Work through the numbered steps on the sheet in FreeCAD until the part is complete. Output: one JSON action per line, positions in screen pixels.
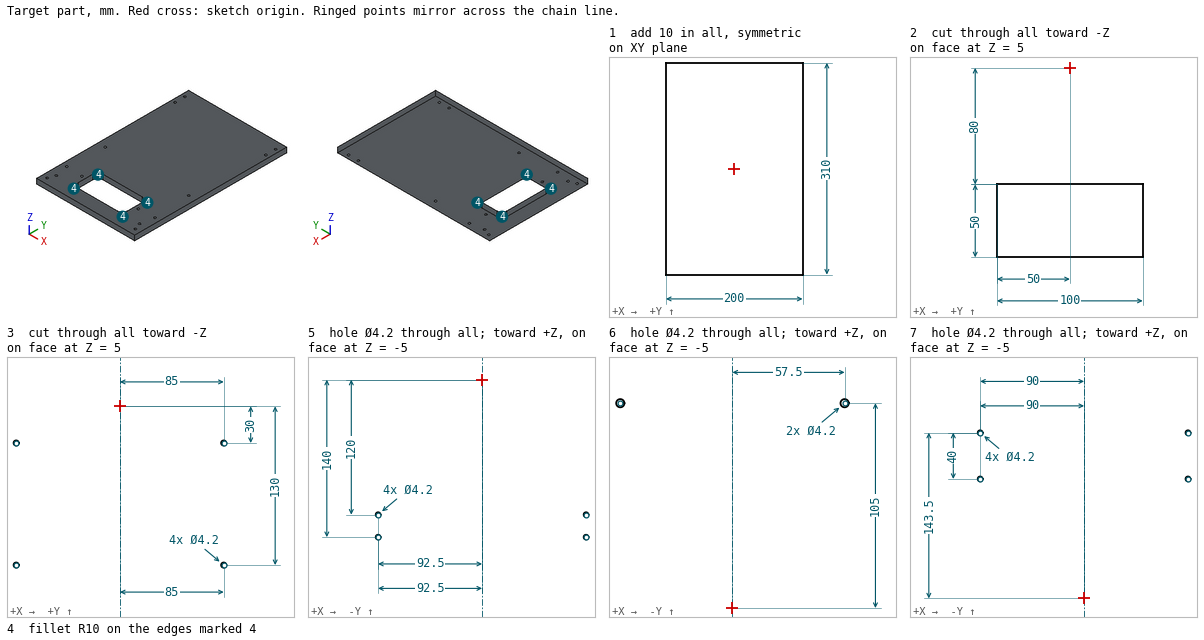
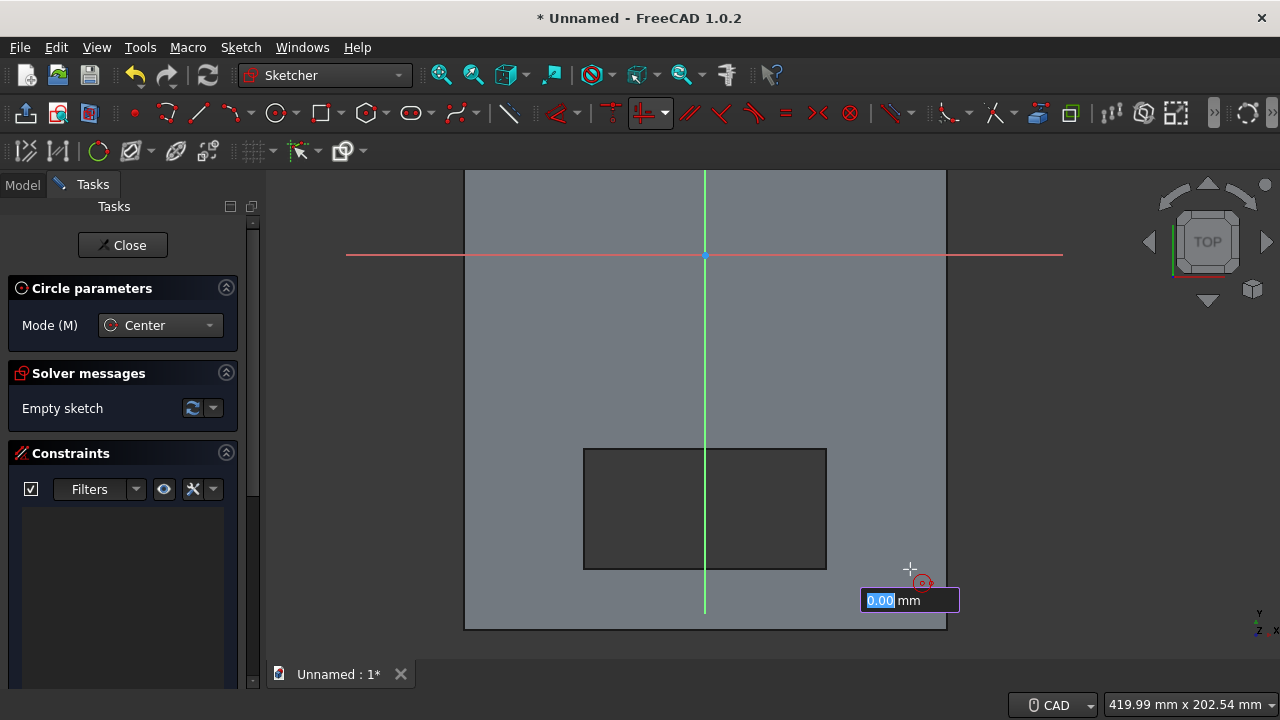
{"action": "scroll", "coordinate": [914, 566], "scroll_direction": "up", "scroll_amount": 6}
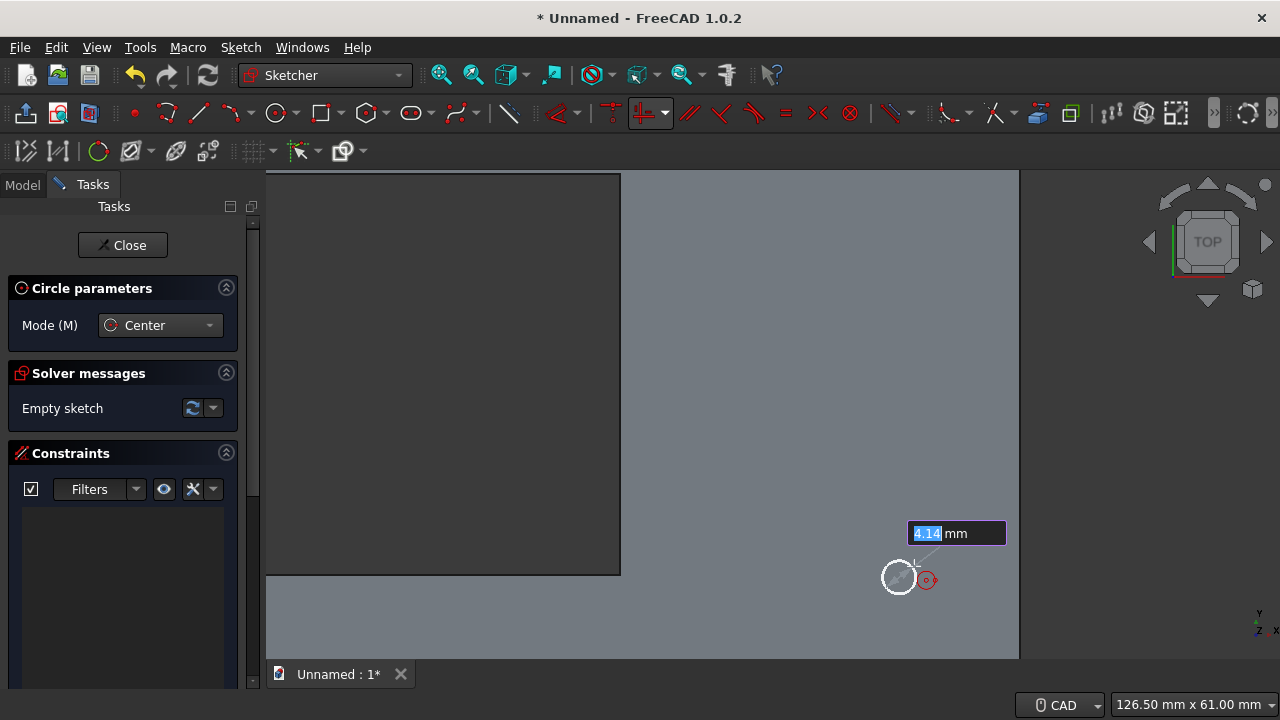
{"action": "left_click", "coordinate": [912, 563]}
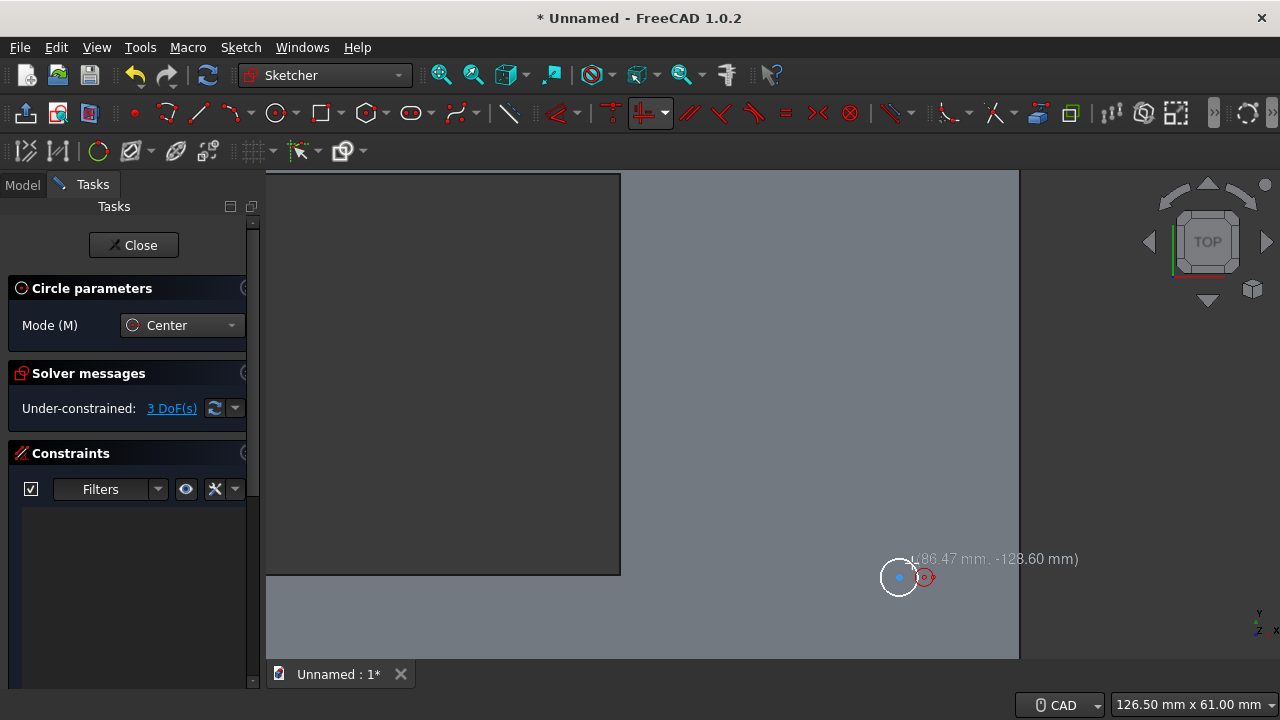
{"action": "scroll", "coordinate": [914, 566], "scroll_direction": "down", "scroll_amount": 6}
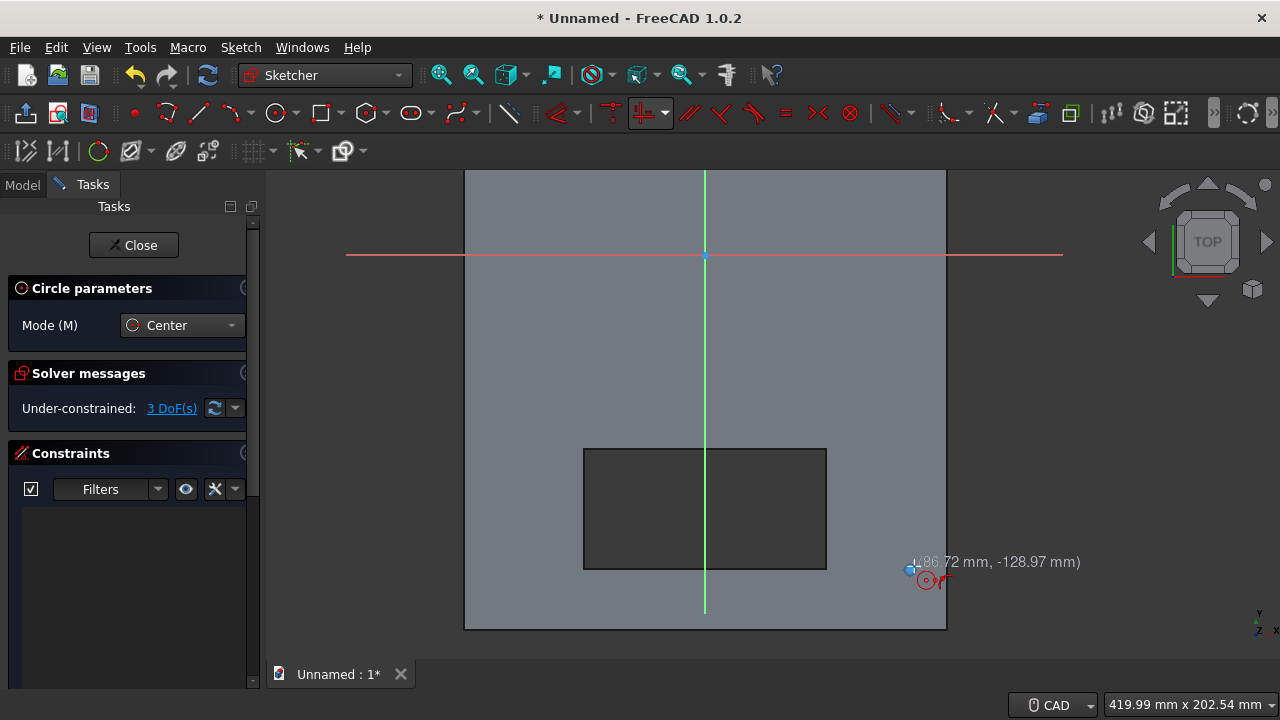
{"action": "scroll", "coordinate": [910, 328], "scroll_direction": "up", "scroll_amount": 8}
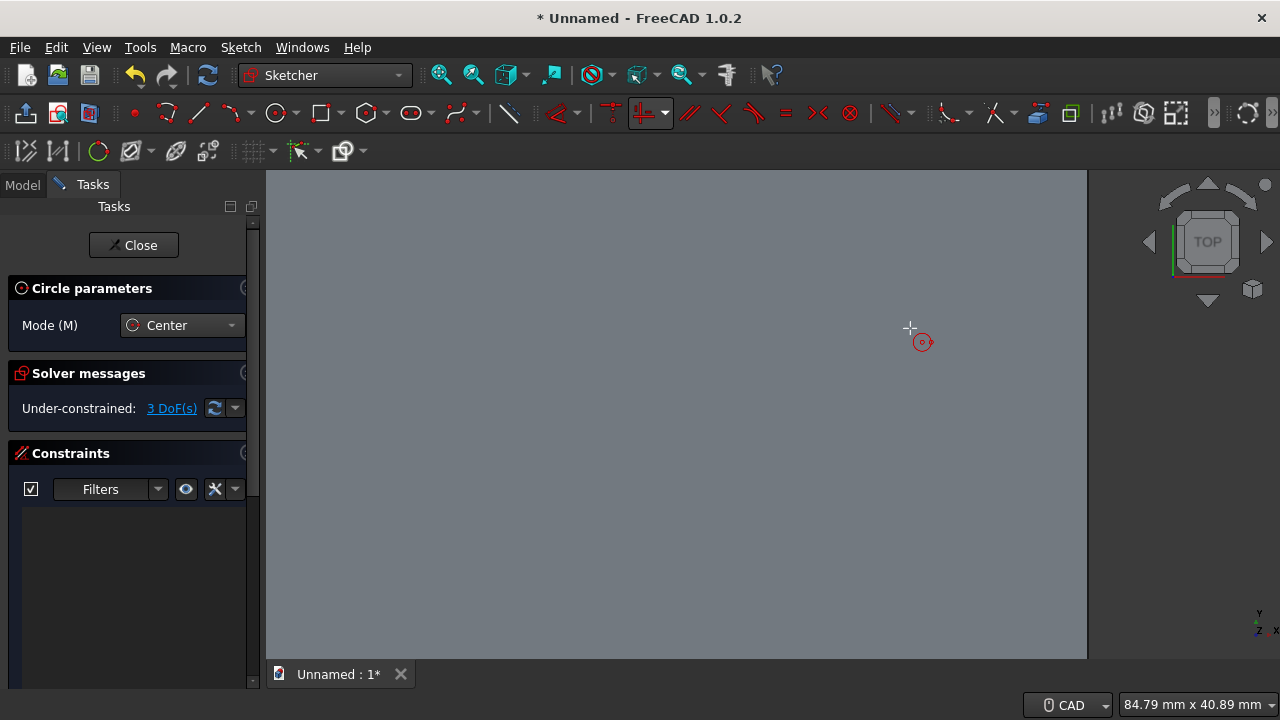
{"action": "scroll", "coordinate": [910, 328], "scroll_direction": "down", "scroll_amount": 8}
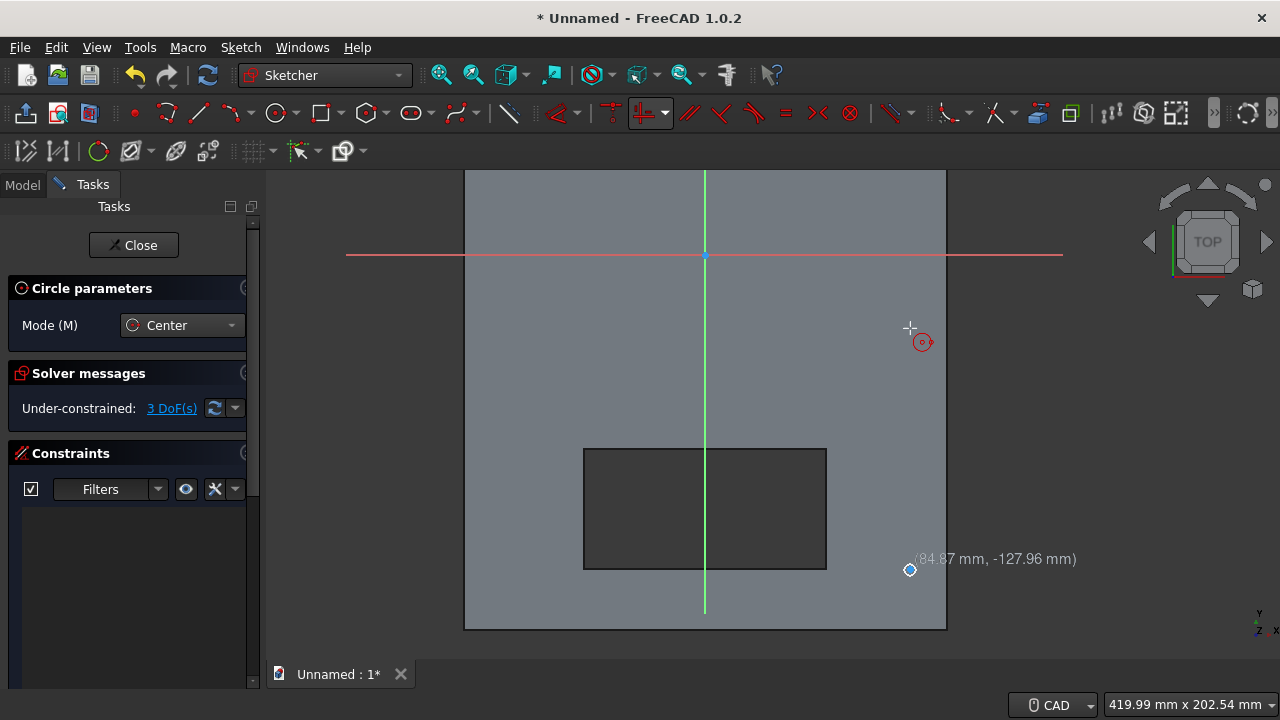
{"action": "left_click", "coordinate": [910, 328]}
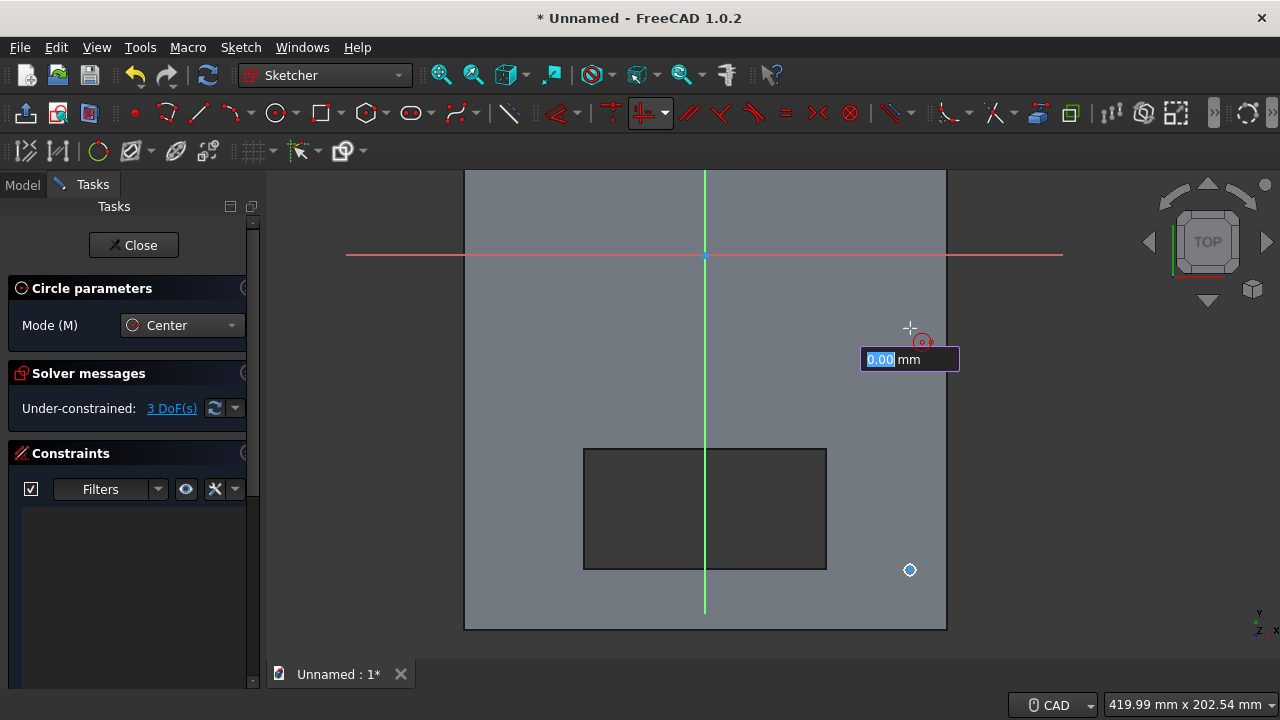
{"action": "scroll", "coordinate": [914, 324], "scroll_direction": "up", "scroll_amount": 6}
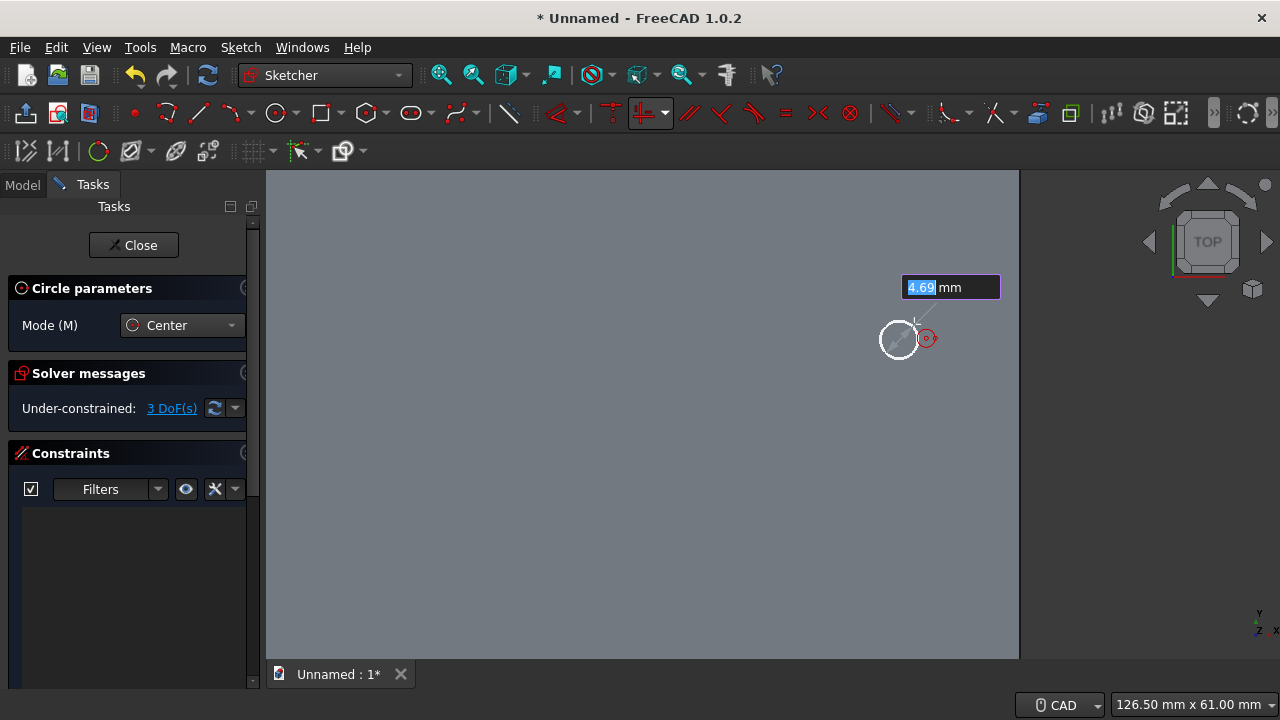
{"action": "left_click", "coordinate": [912, 324]}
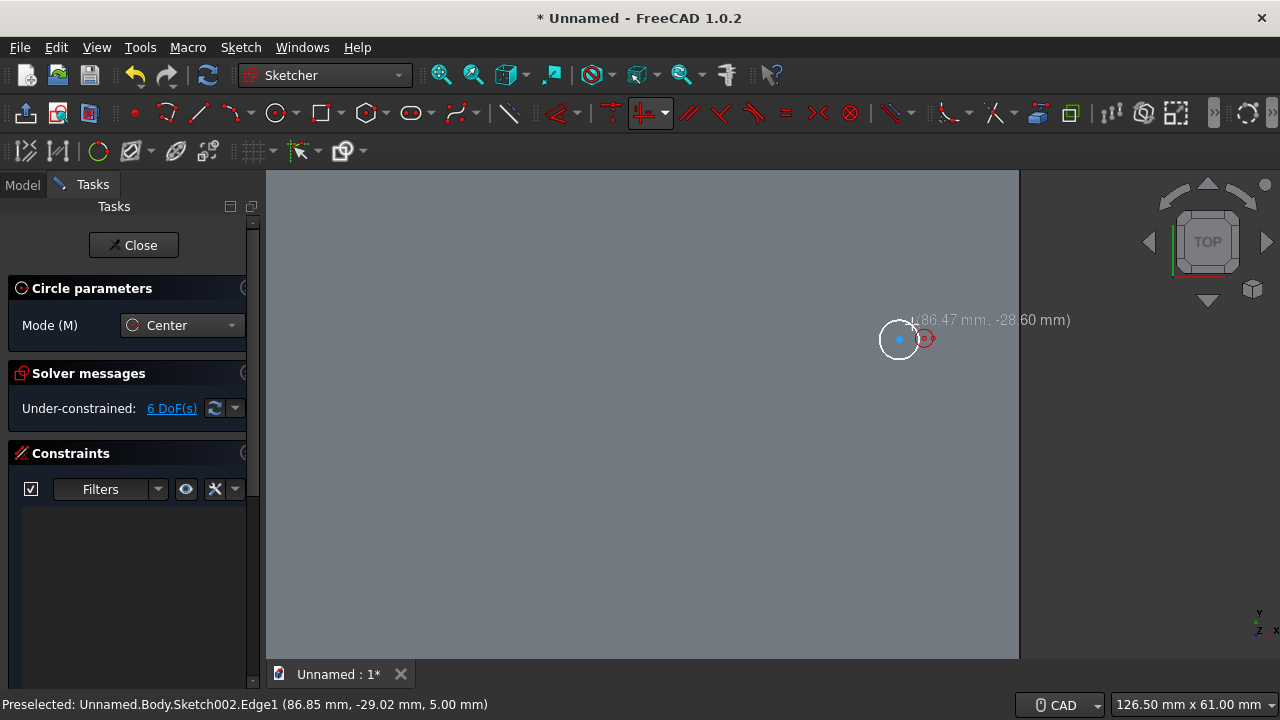
{"action": "scroll", "coordinate": [914, 324], "scroll_direction": "down", "scroll_amount": 6}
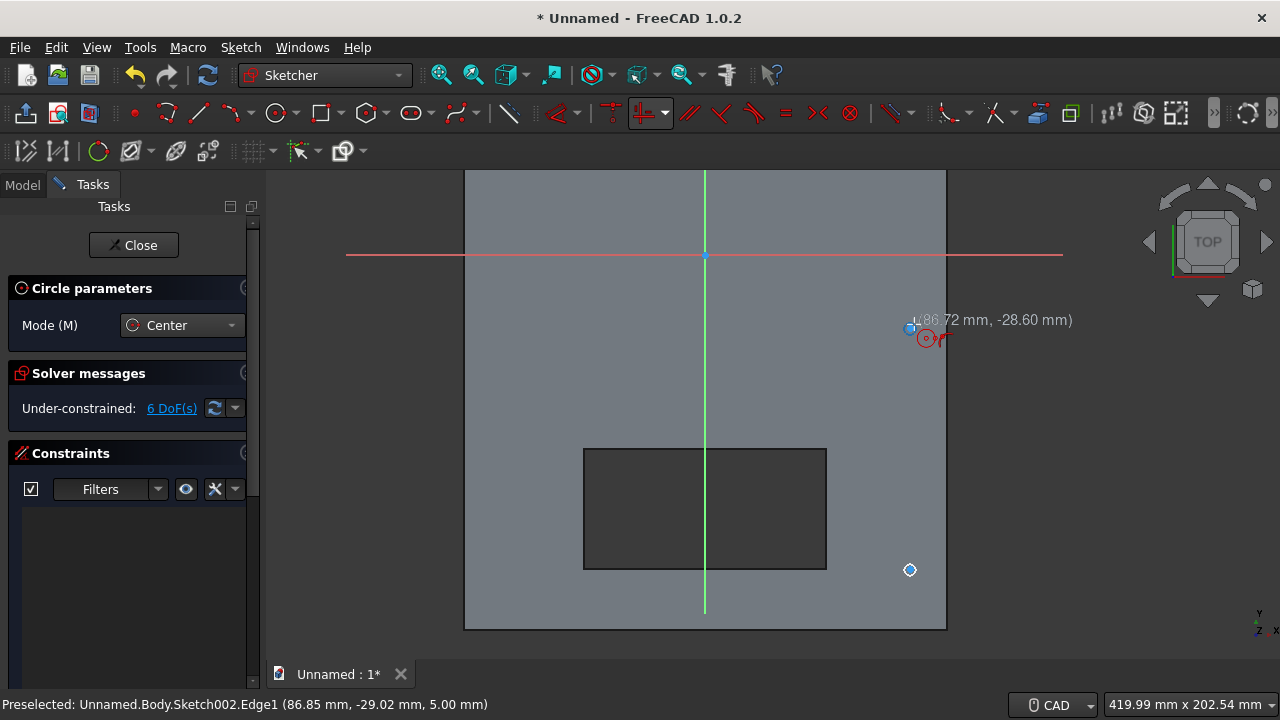
{"action": "scroll", "coordinate": [500, 328], "scroll_direction": "up", "scroll_amount": 8}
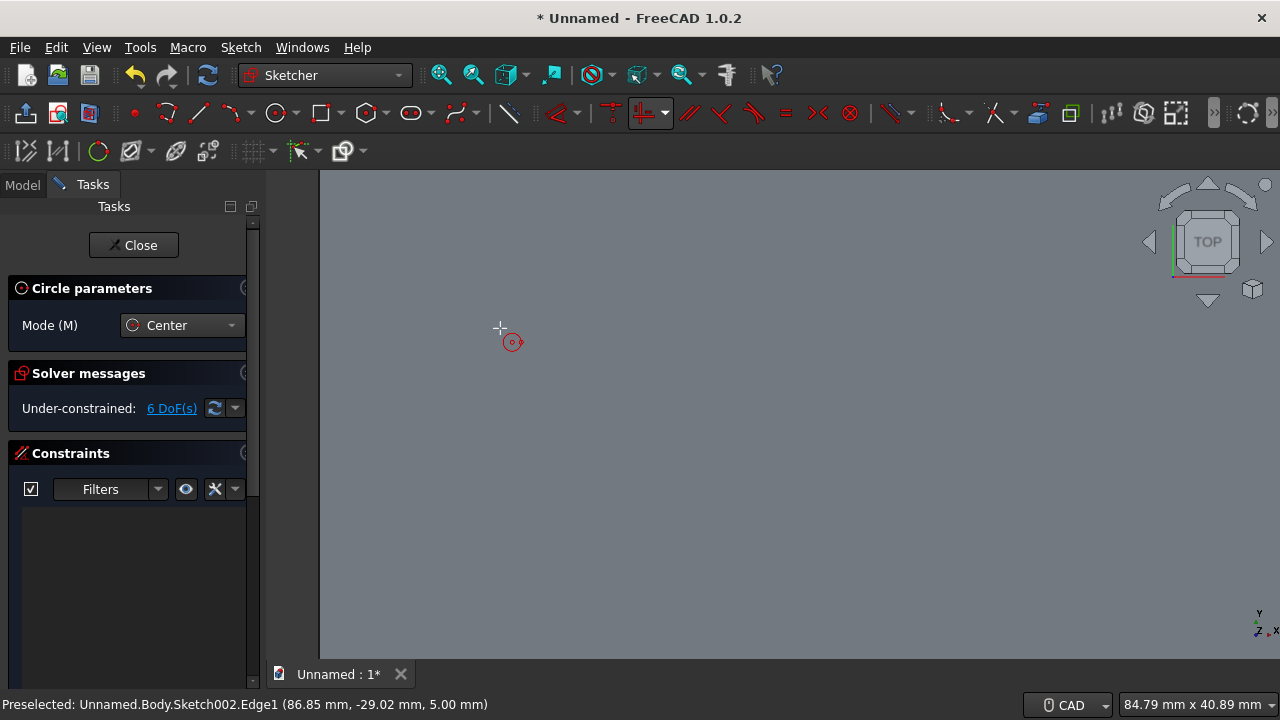
{"action": "scroll", "coordinate": [499, 328], "scroll_direction": "down", "scroll_amount": 8}